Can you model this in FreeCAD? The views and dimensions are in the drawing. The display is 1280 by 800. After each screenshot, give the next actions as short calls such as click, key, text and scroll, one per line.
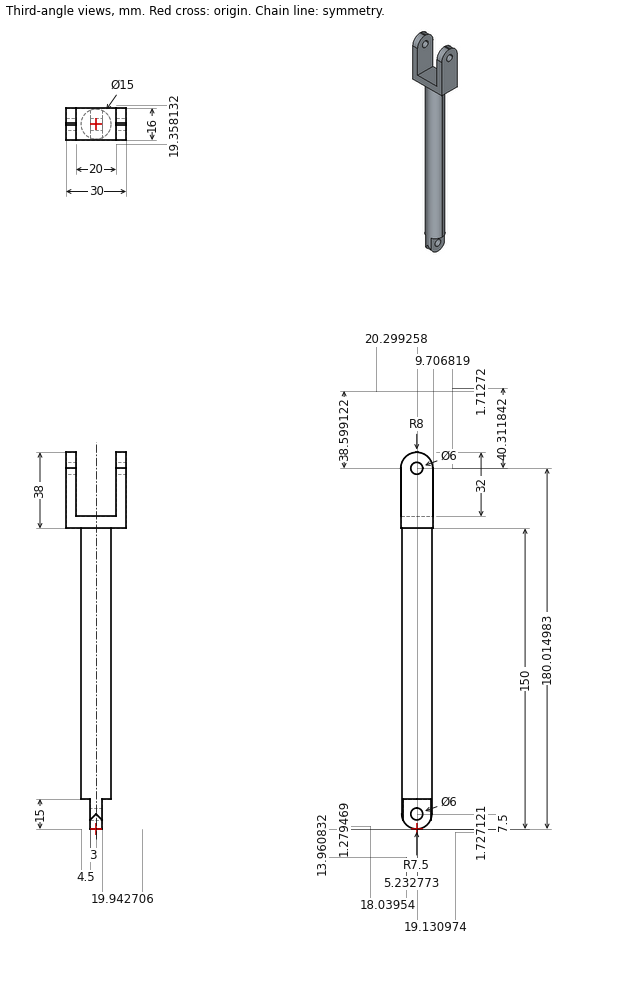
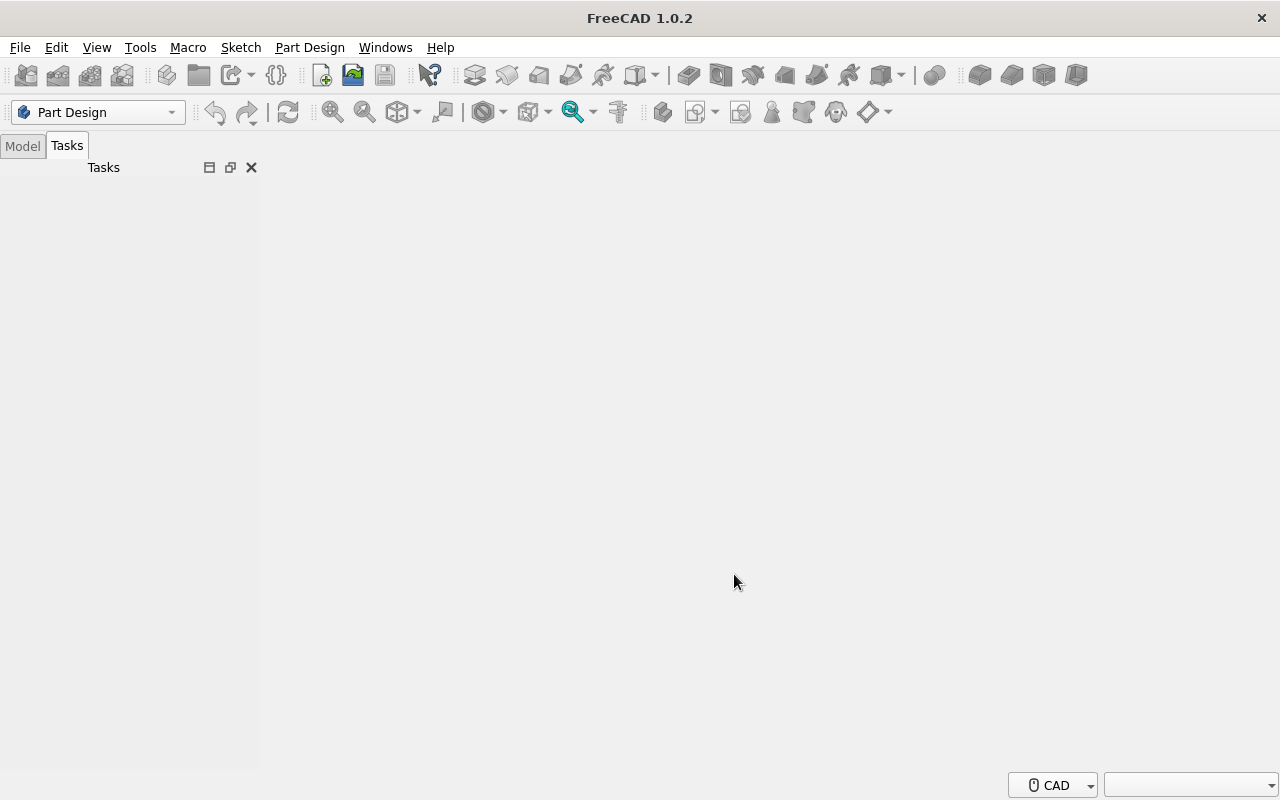
key(ctrl+n)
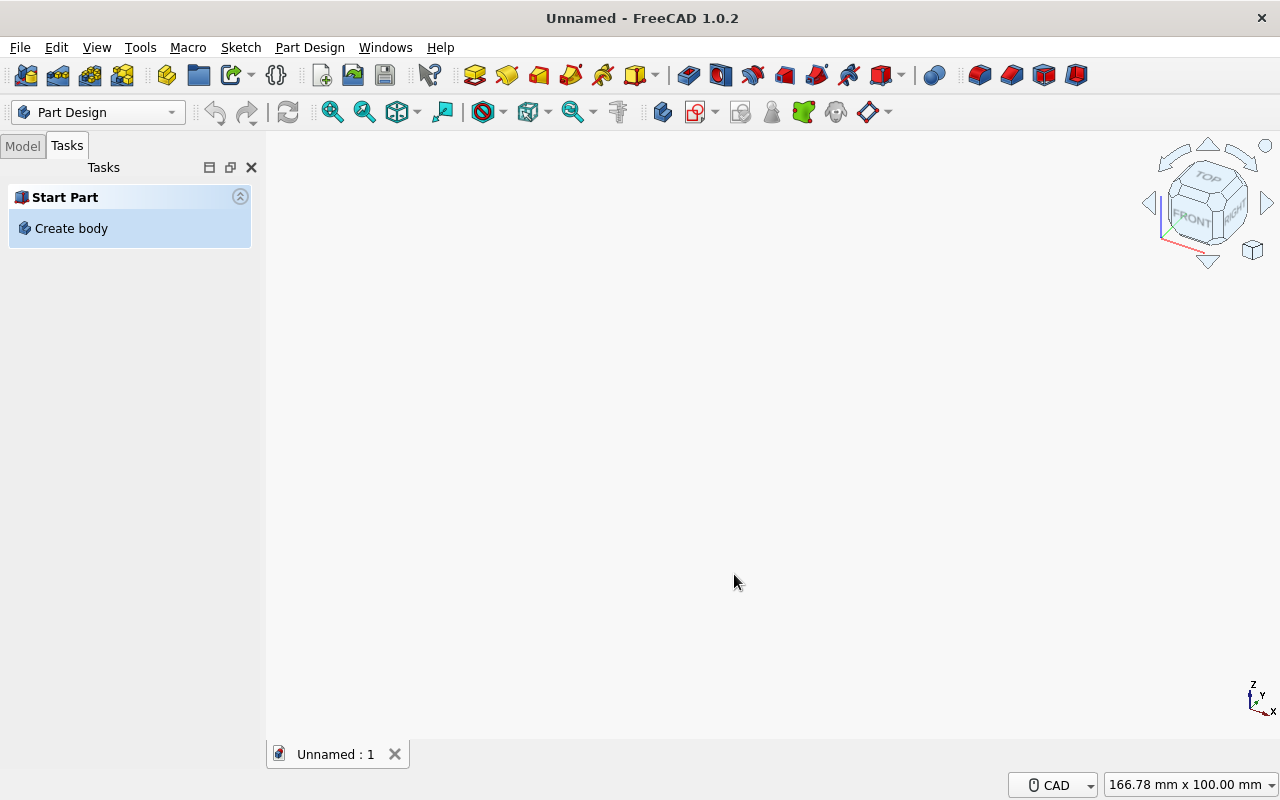
click(696, 112)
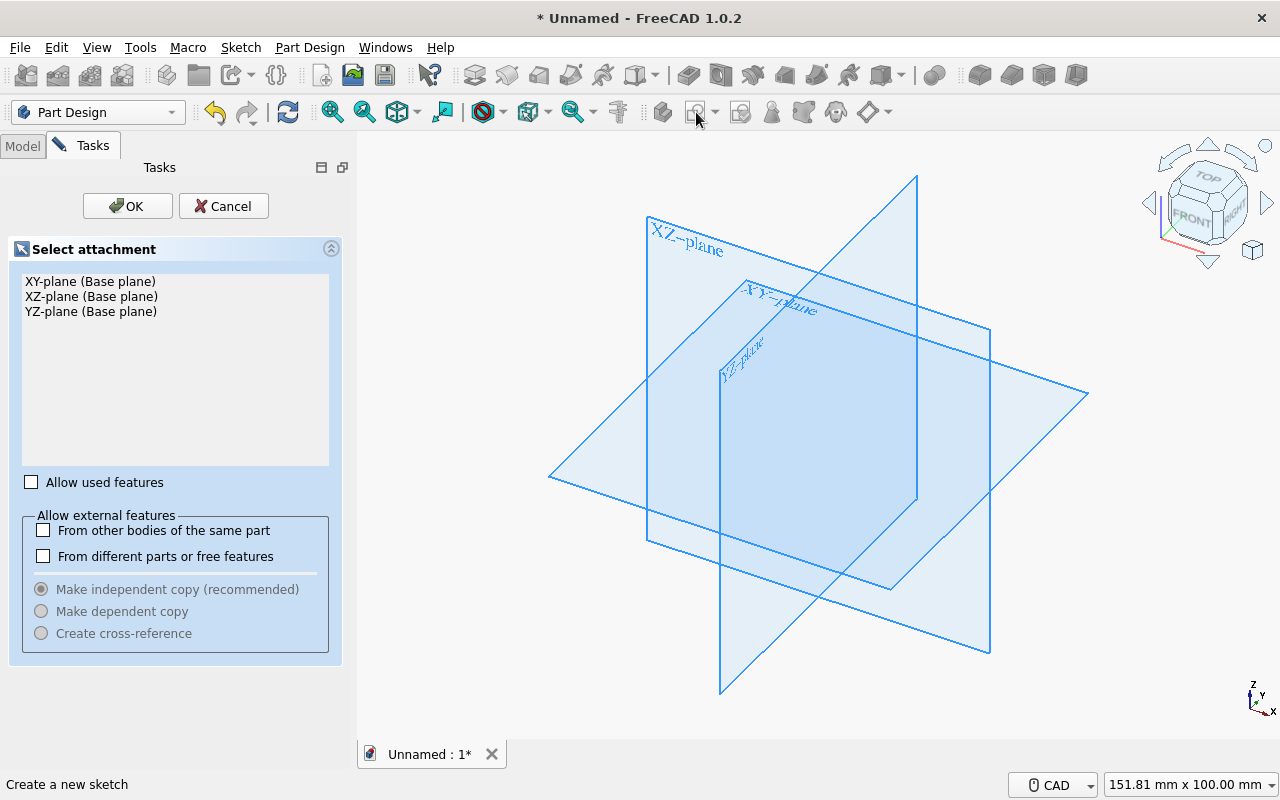
click(82, 282)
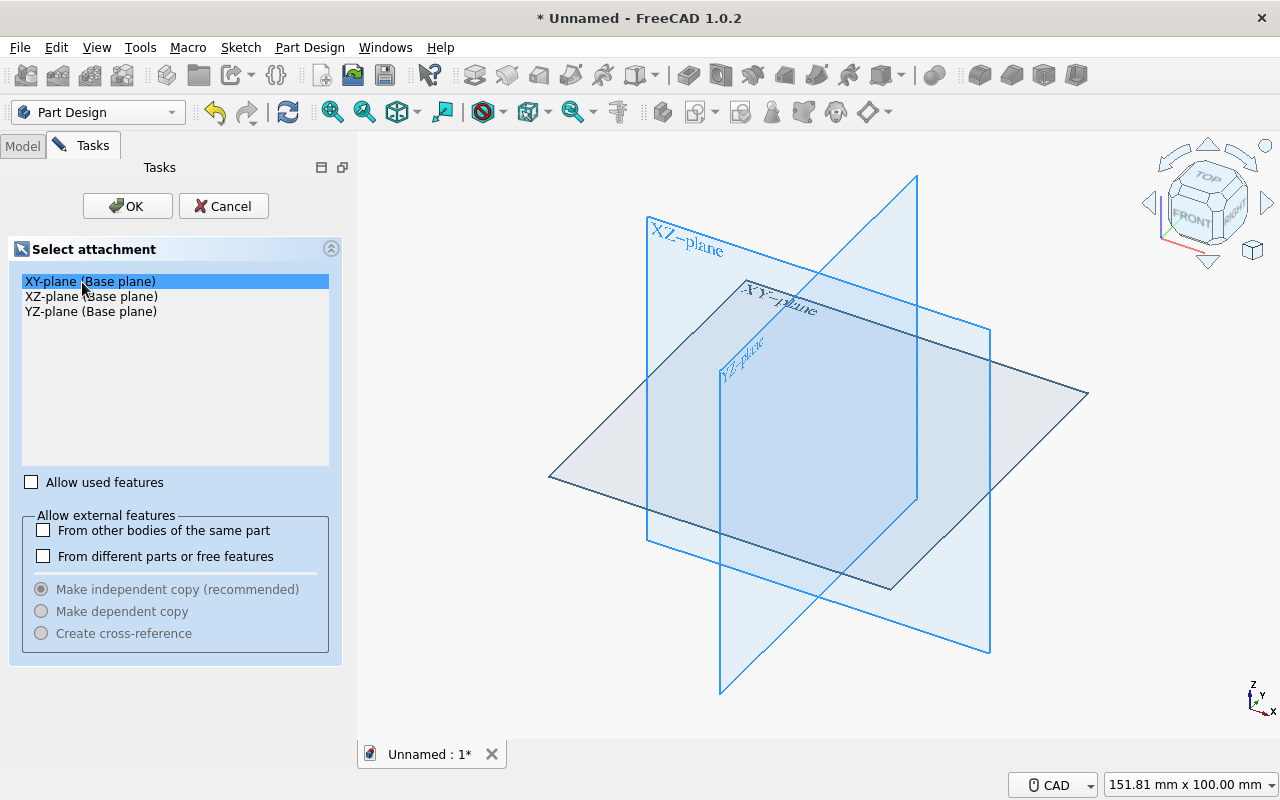
click(128, 206)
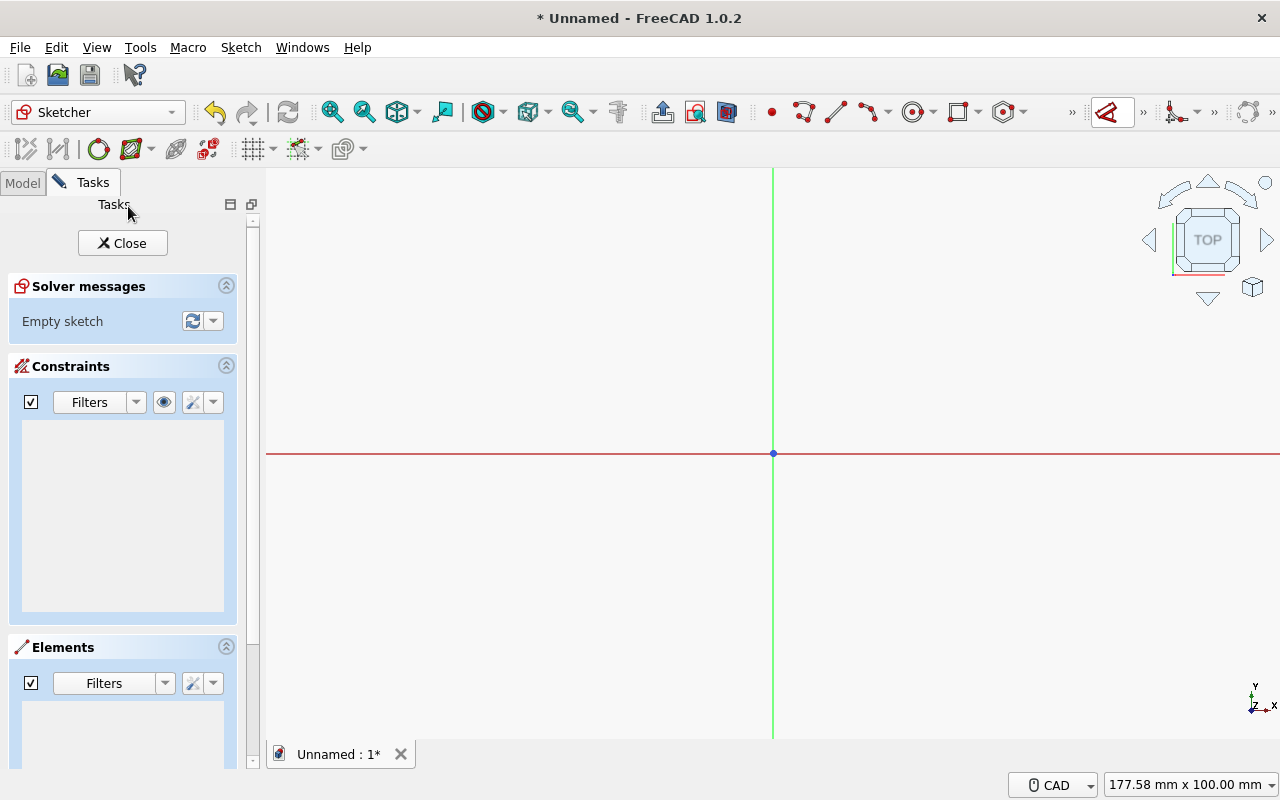
scroll(795, 454, up, 7)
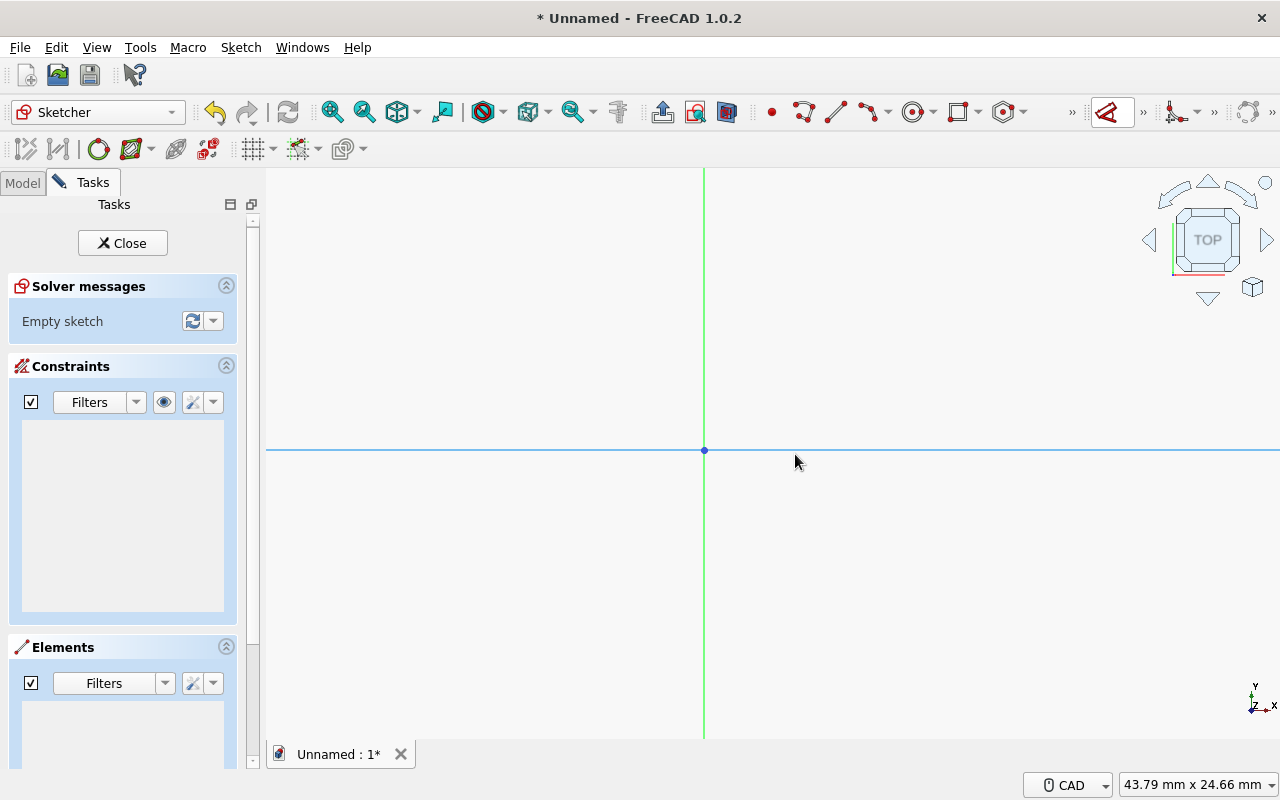
click(914, 112)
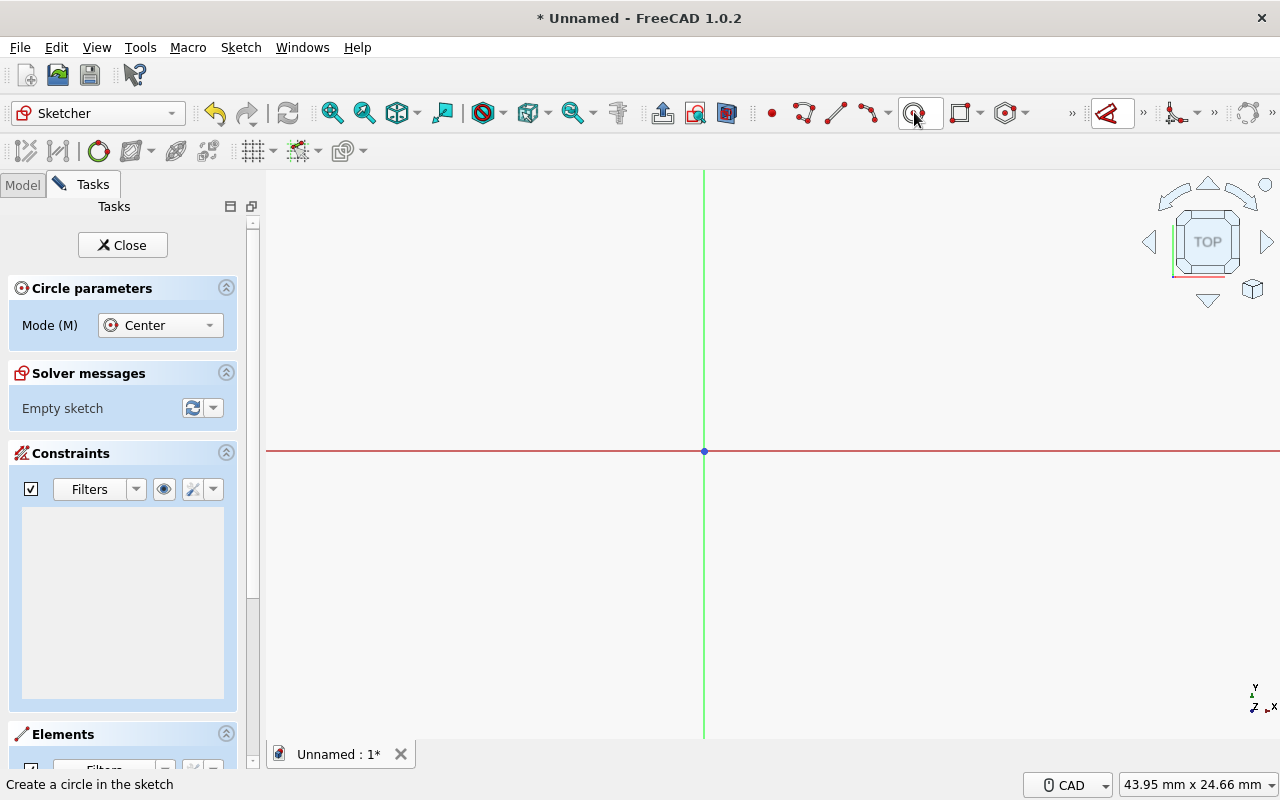
click(704, 451)
move(827, 329)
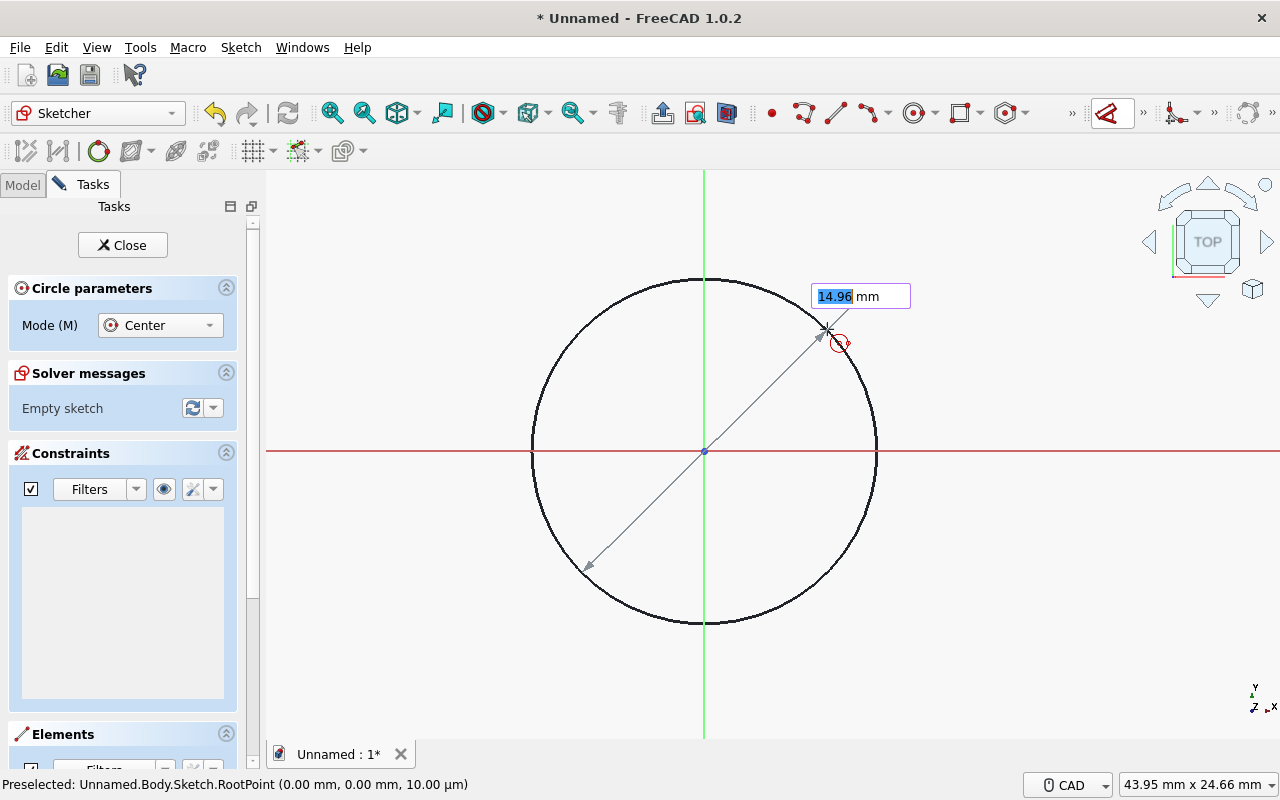
text(15)
key(Return)
key(Escape)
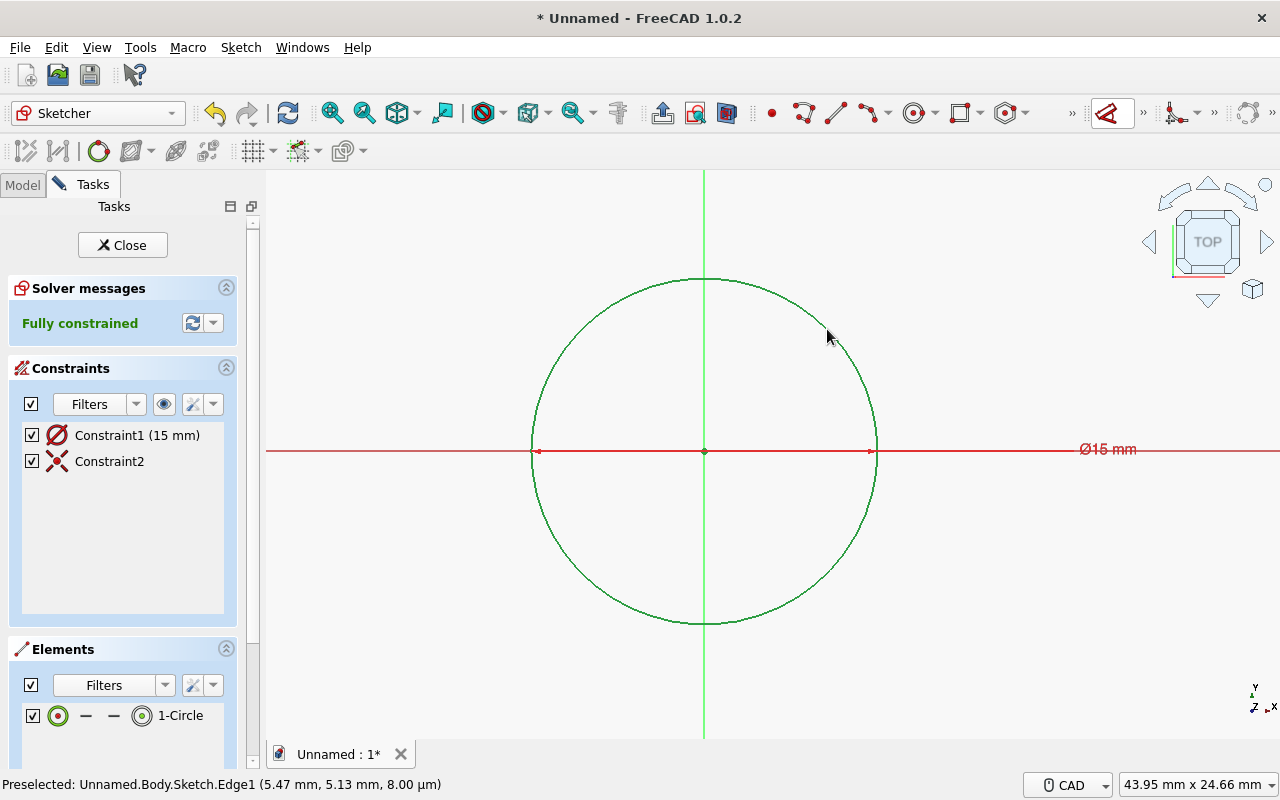
click(123, 245)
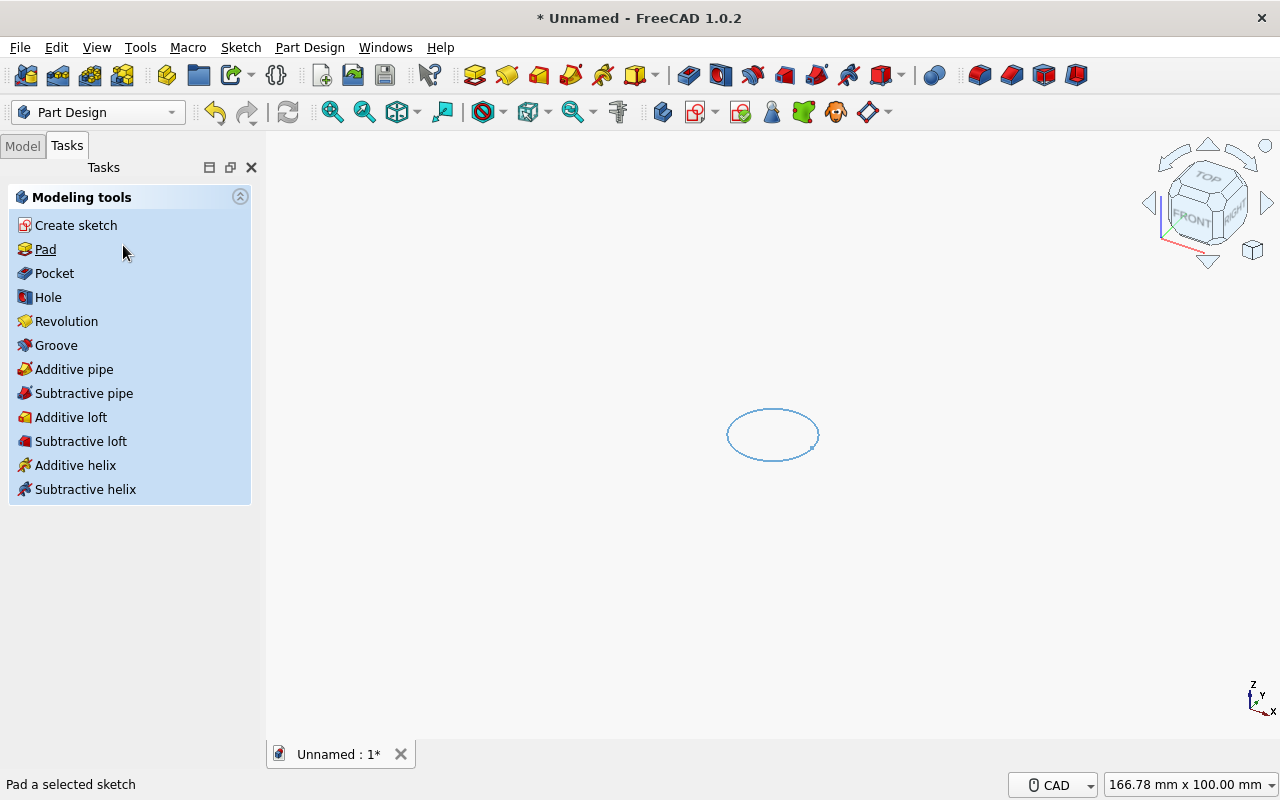
click(476, 76)